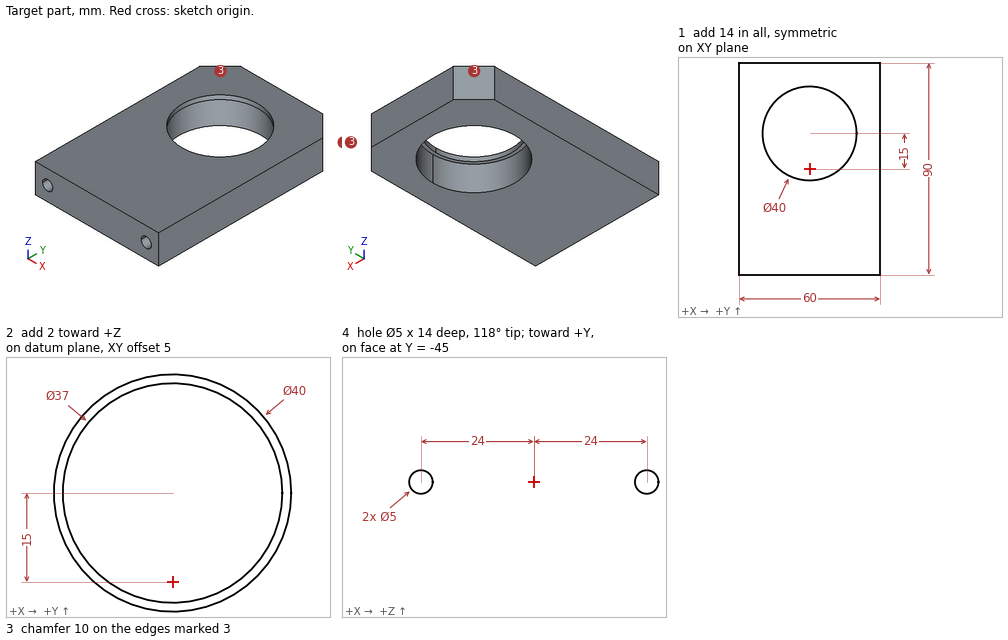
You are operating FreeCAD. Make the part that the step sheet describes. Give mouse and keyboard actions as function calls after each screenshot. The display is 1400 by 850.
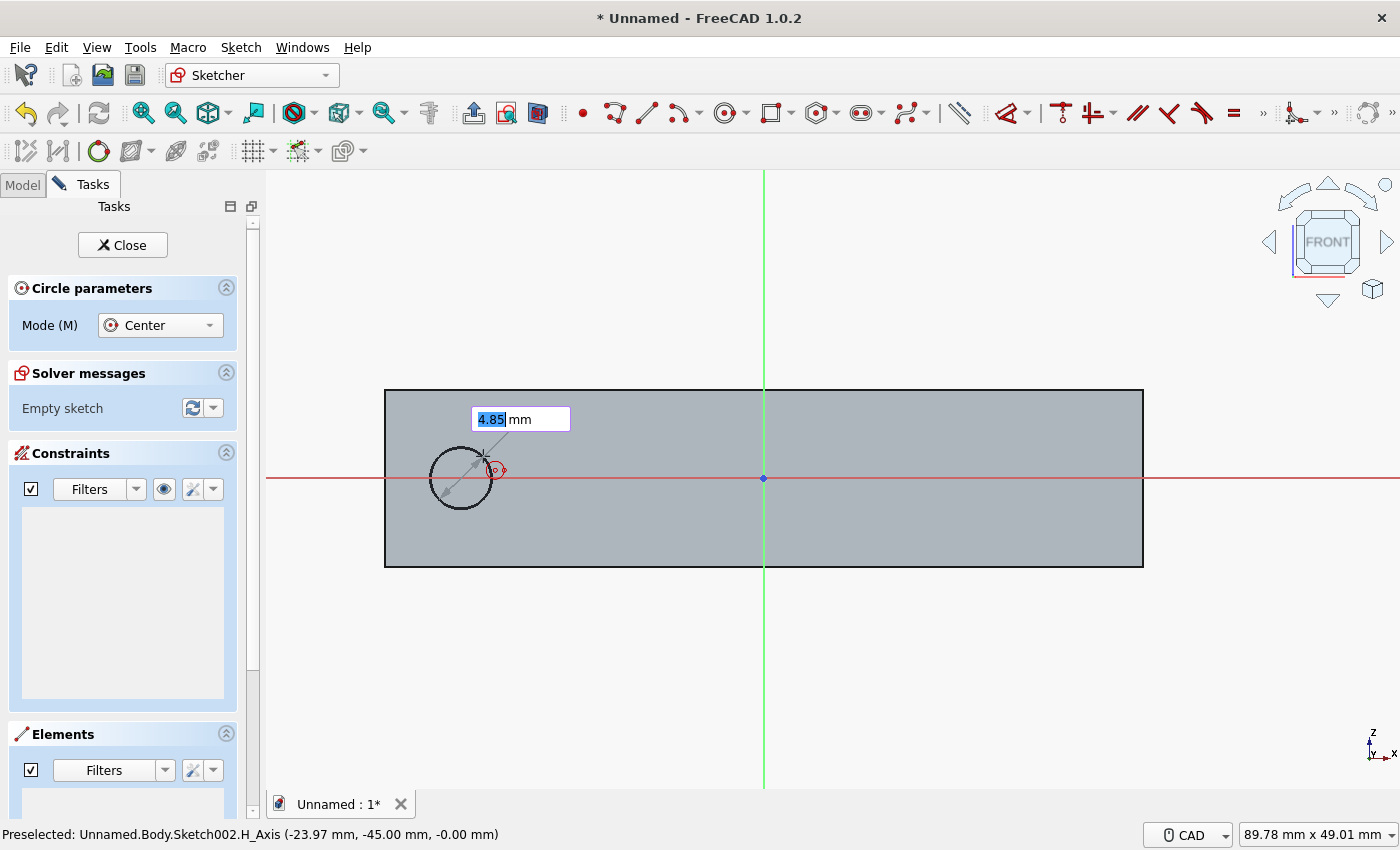
text(5)
key(Return)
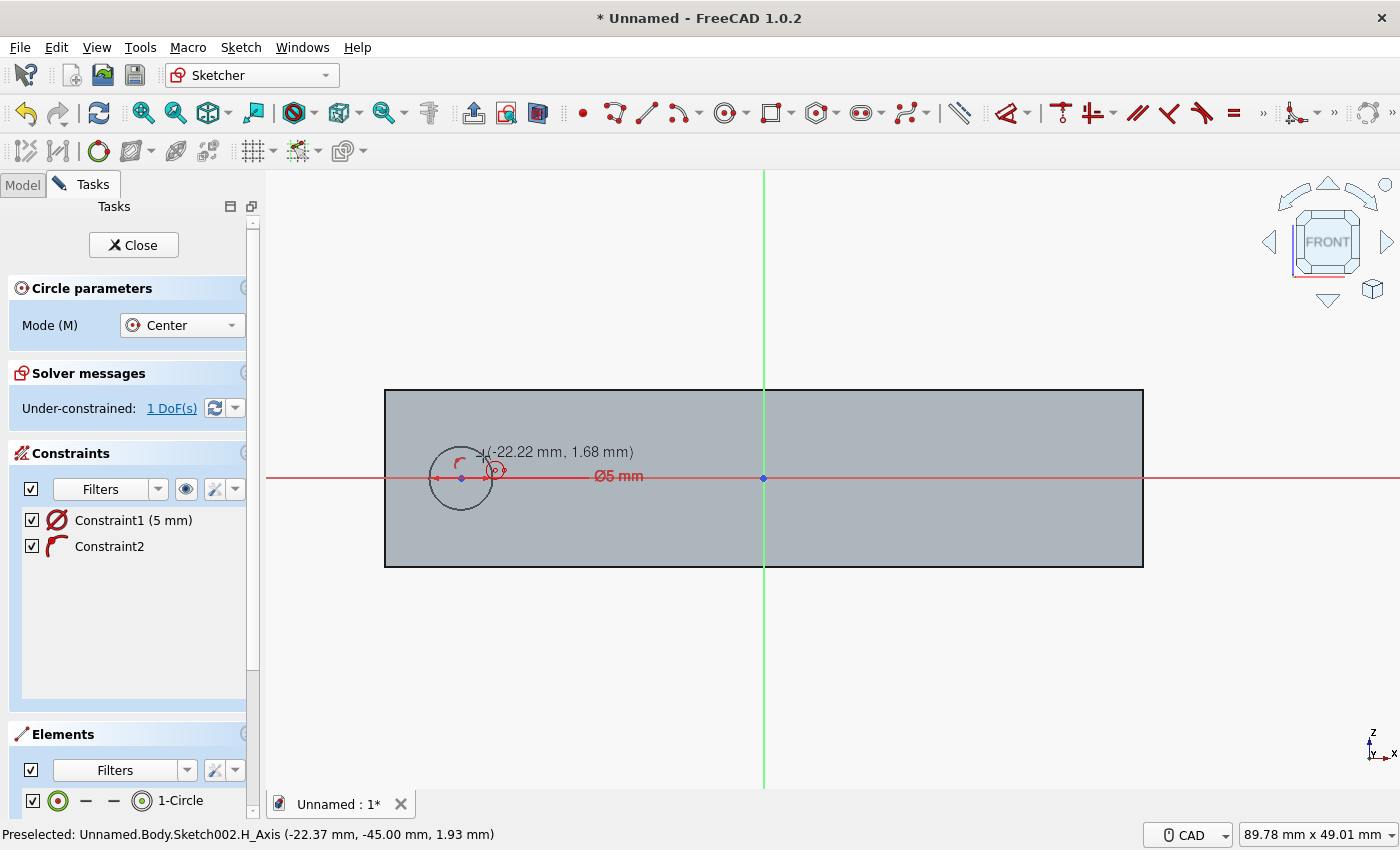
click(1067, 478)
move(1089, 456)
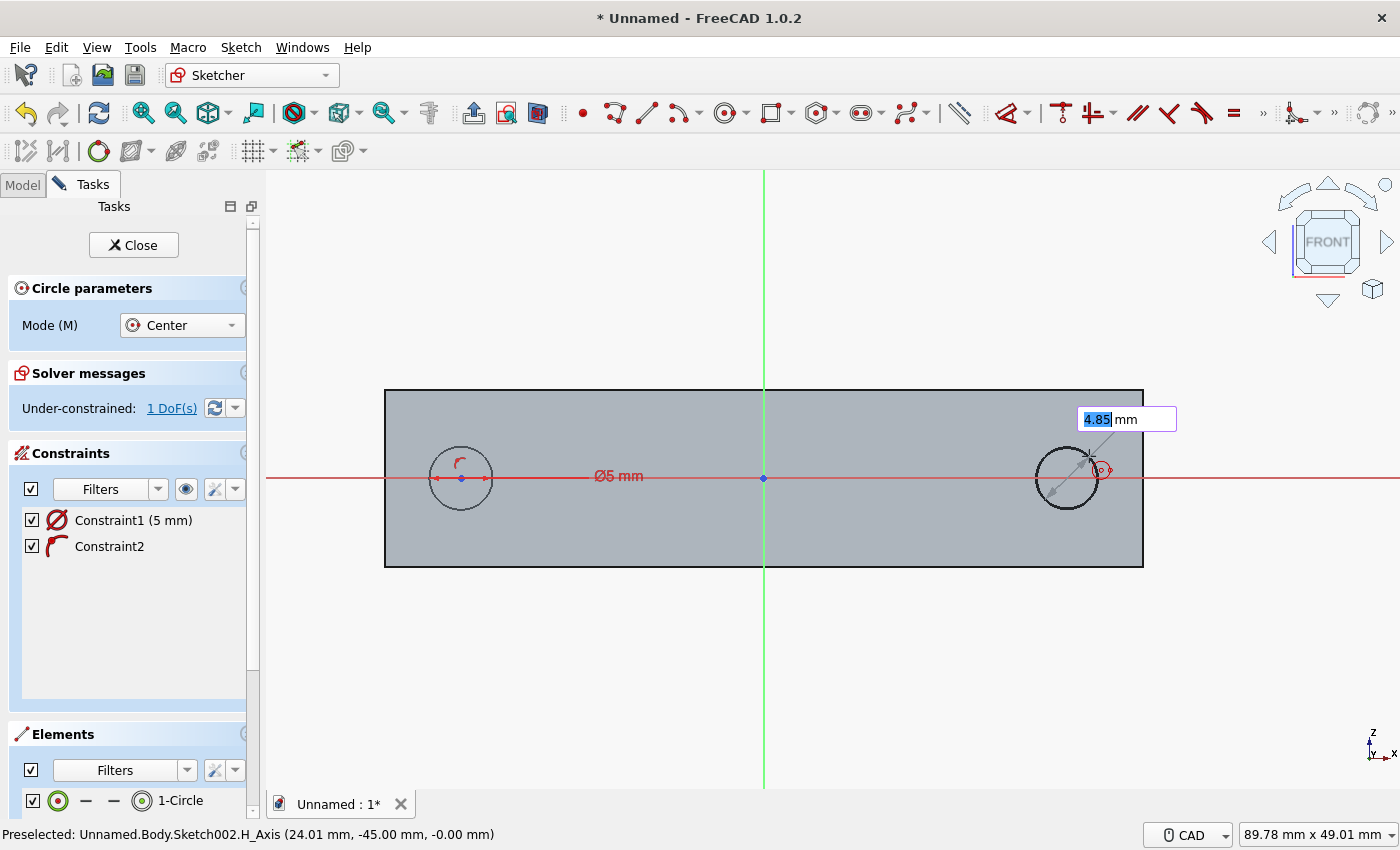
text(5)
key(Return)
key(Escape)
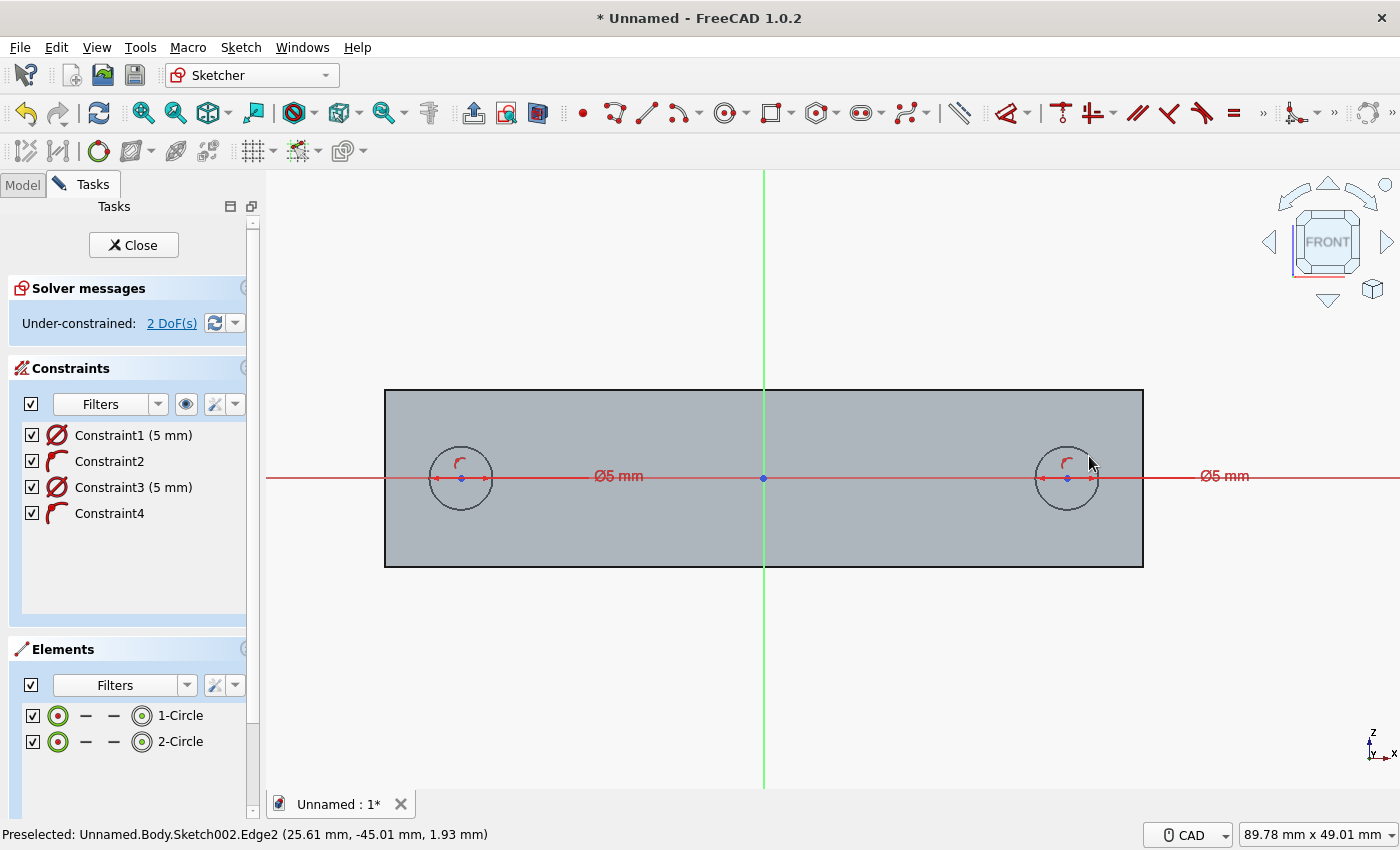
click(1006, 114)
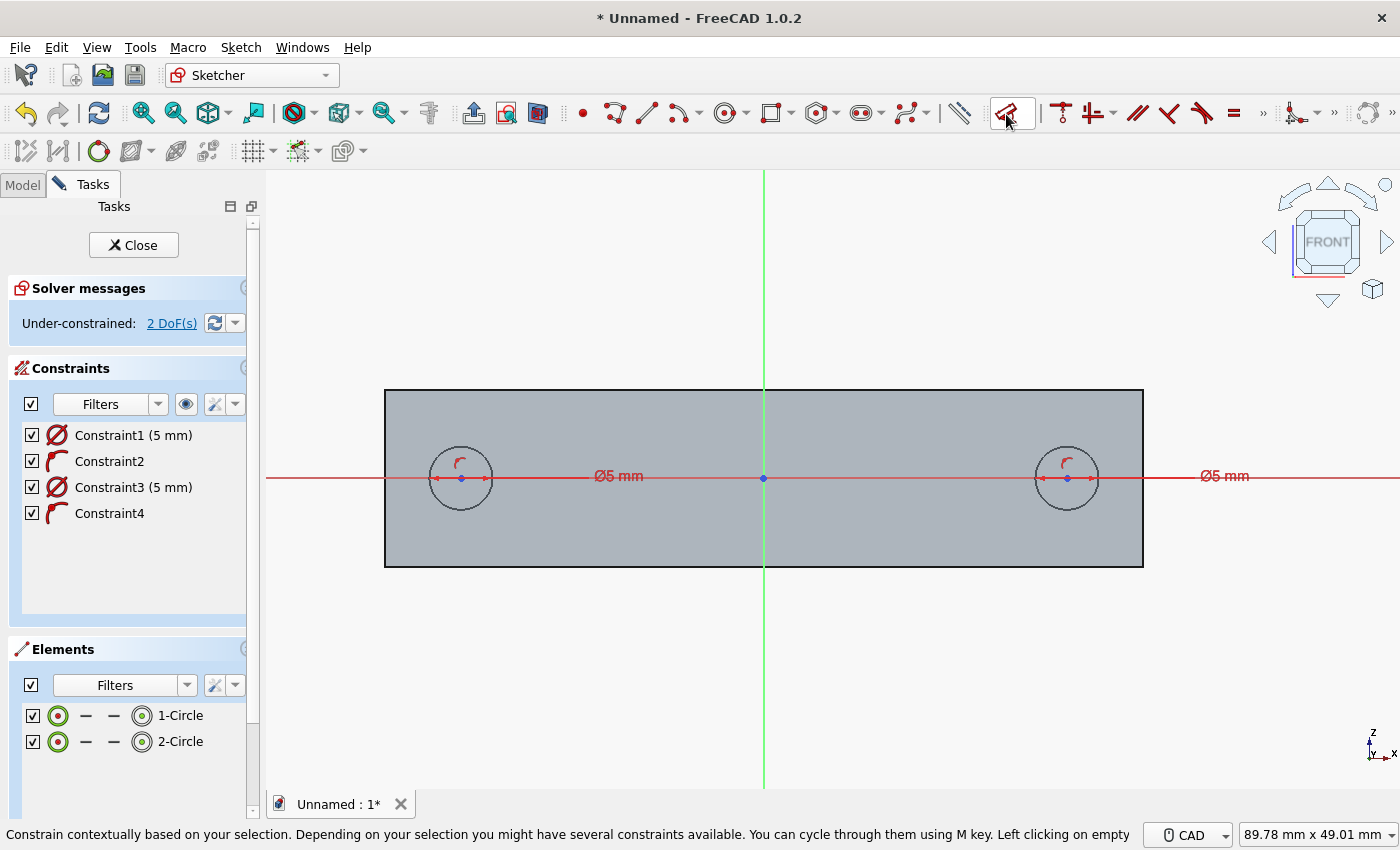
click(461, 478)
click(612, 512)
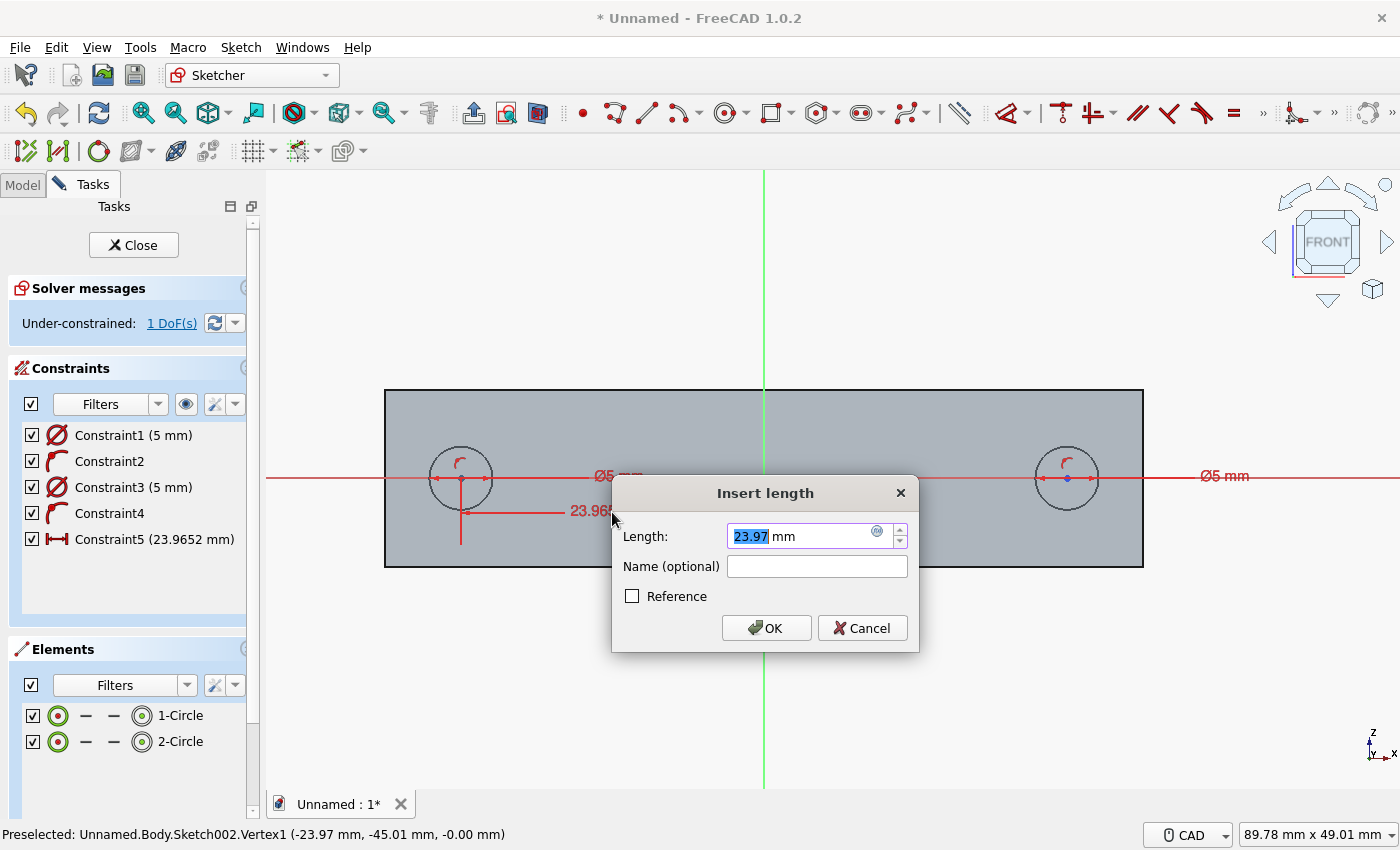
text(24)
key(Return)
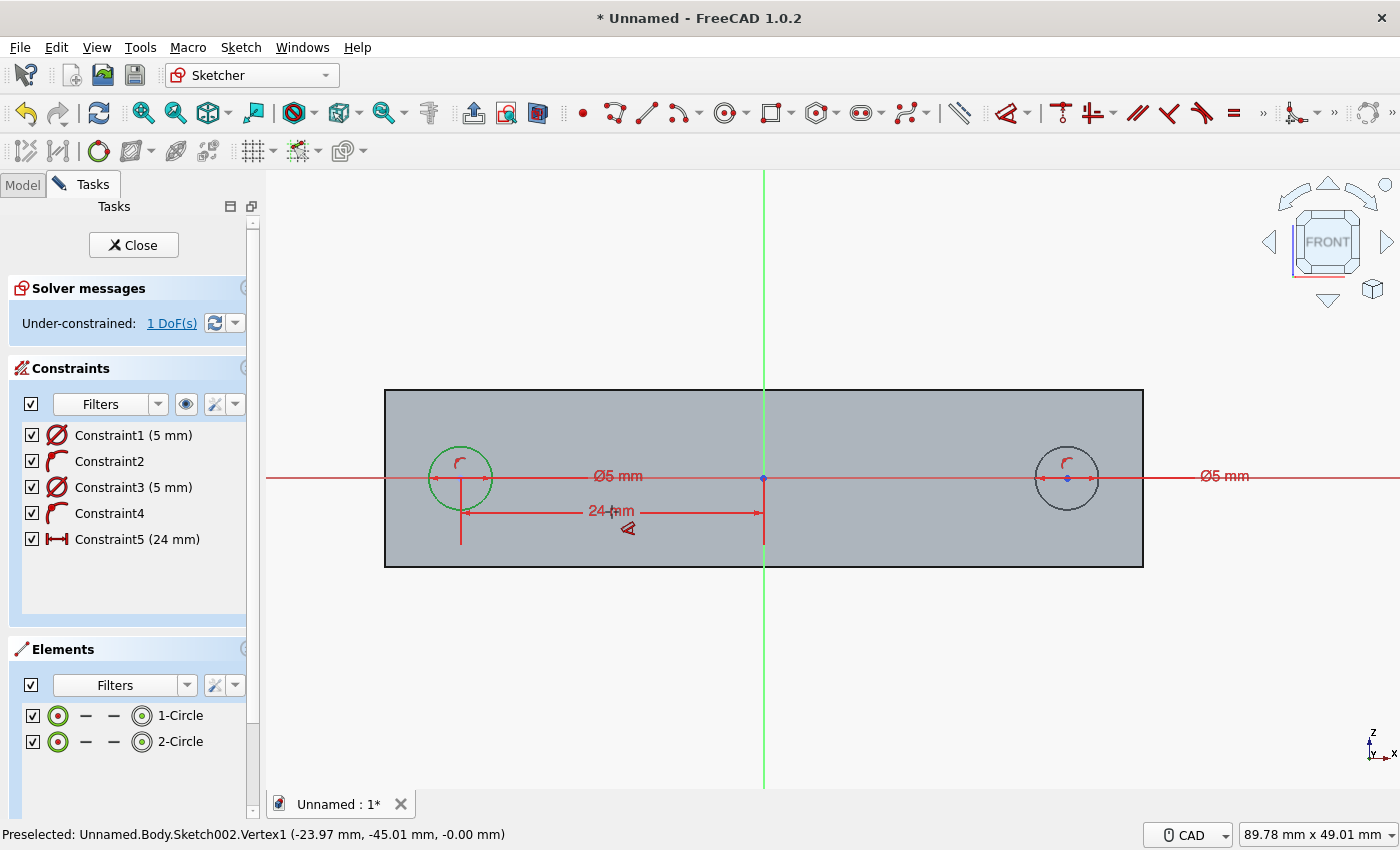
click(1067, 478)
click(915, 512)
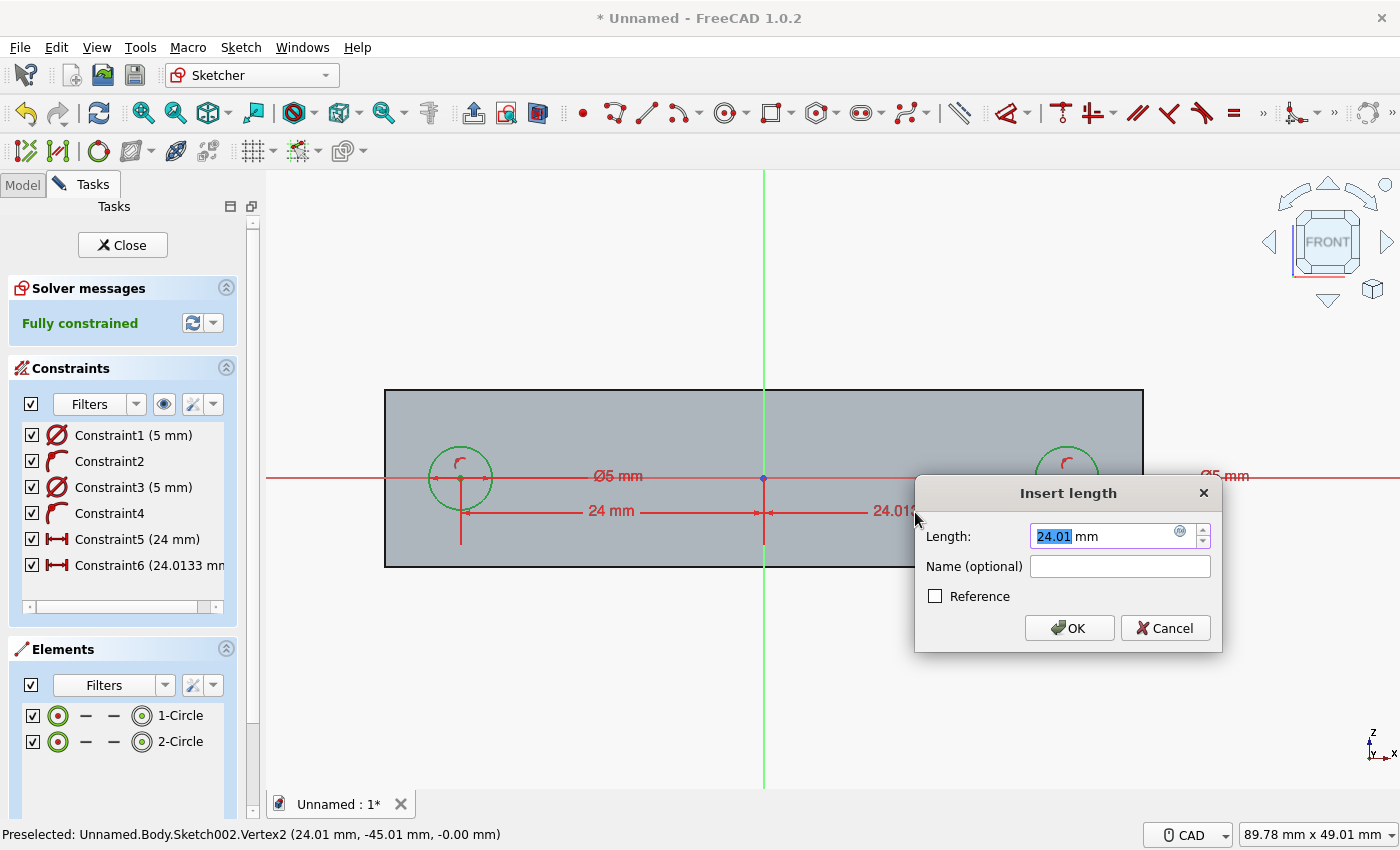
text(24)
key(Return)
key(Escape)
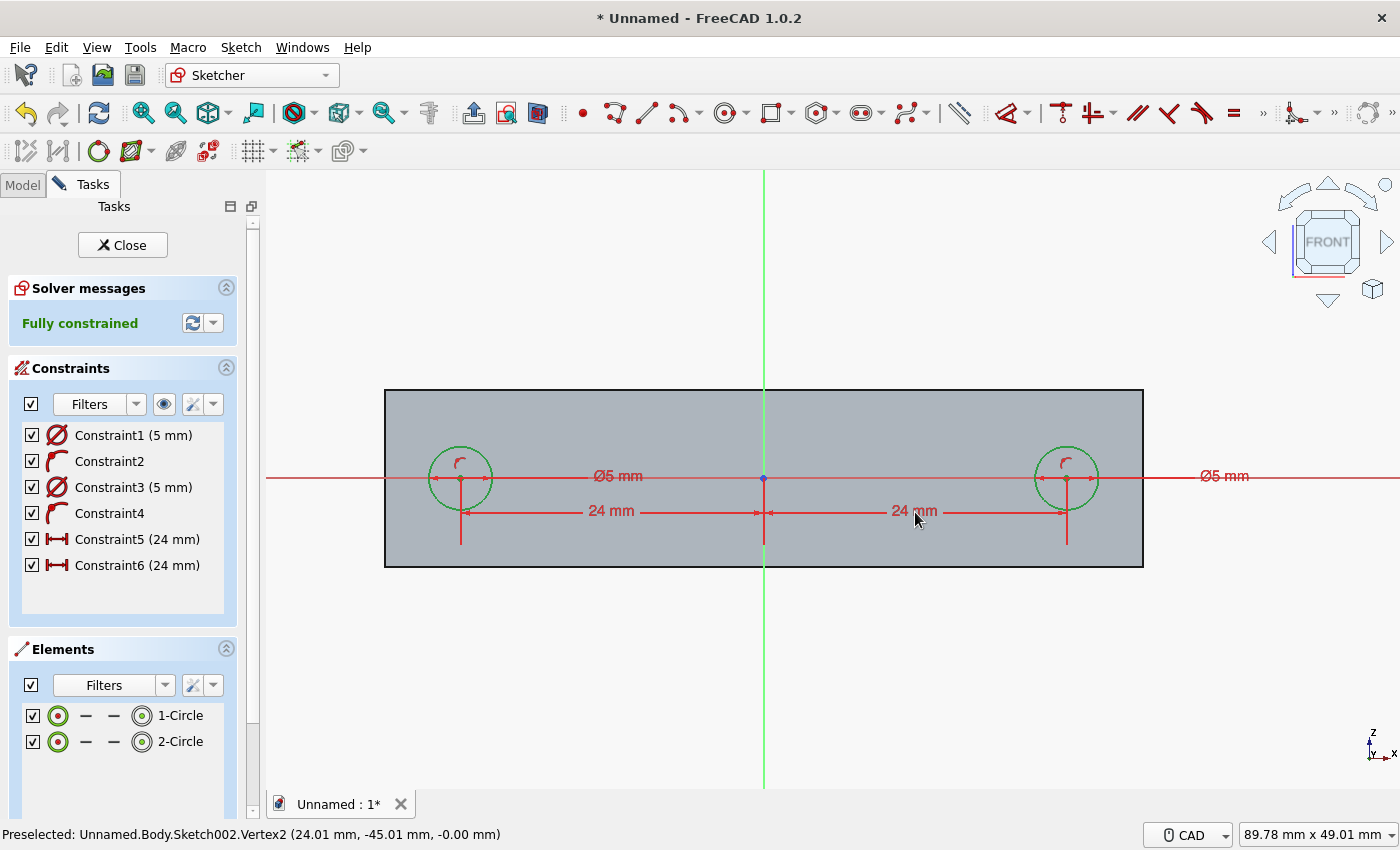
click(123, 245)